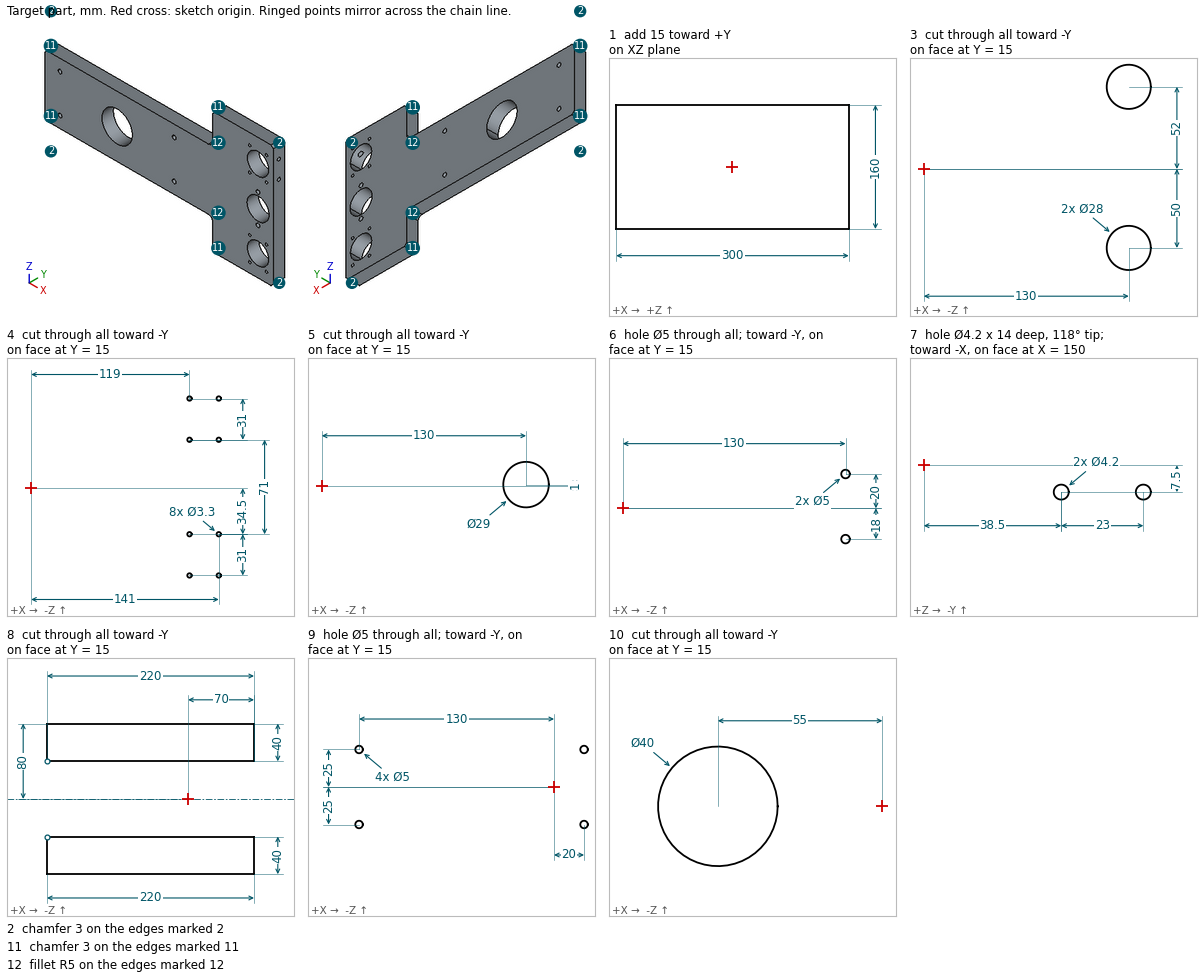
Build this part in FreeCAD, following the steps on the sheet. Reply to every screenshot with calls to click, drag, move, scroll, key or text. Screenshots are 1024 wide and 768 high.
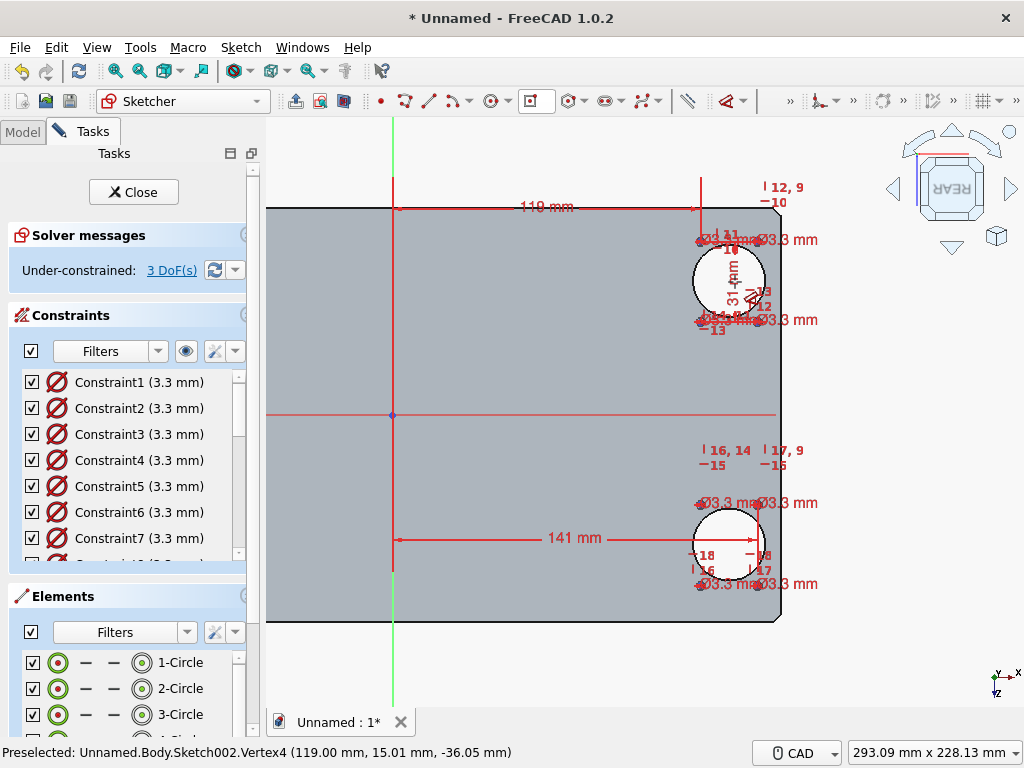
click(758, 505)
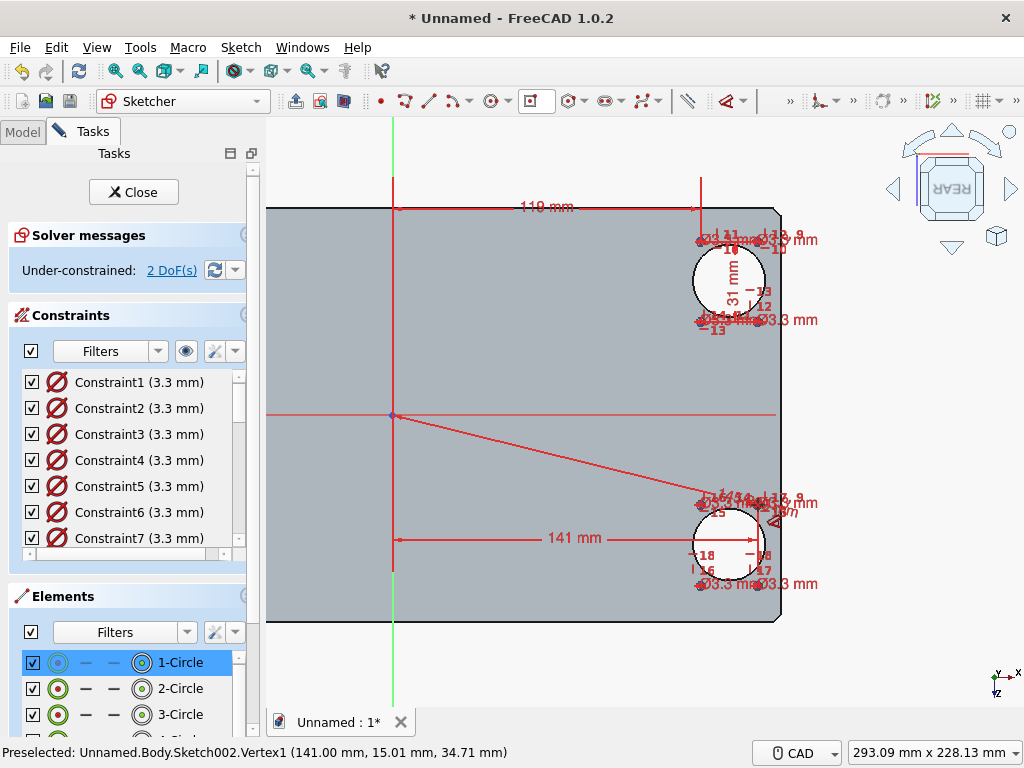
click(701, 322)
click(792, 371)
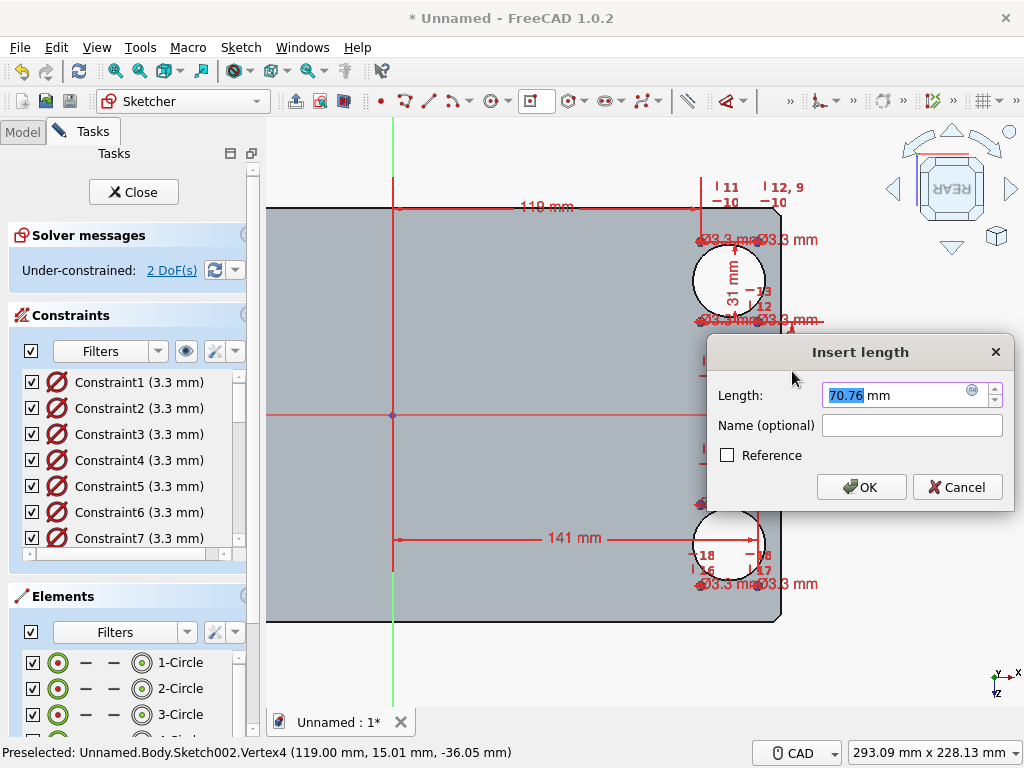
text(71)
key(Return)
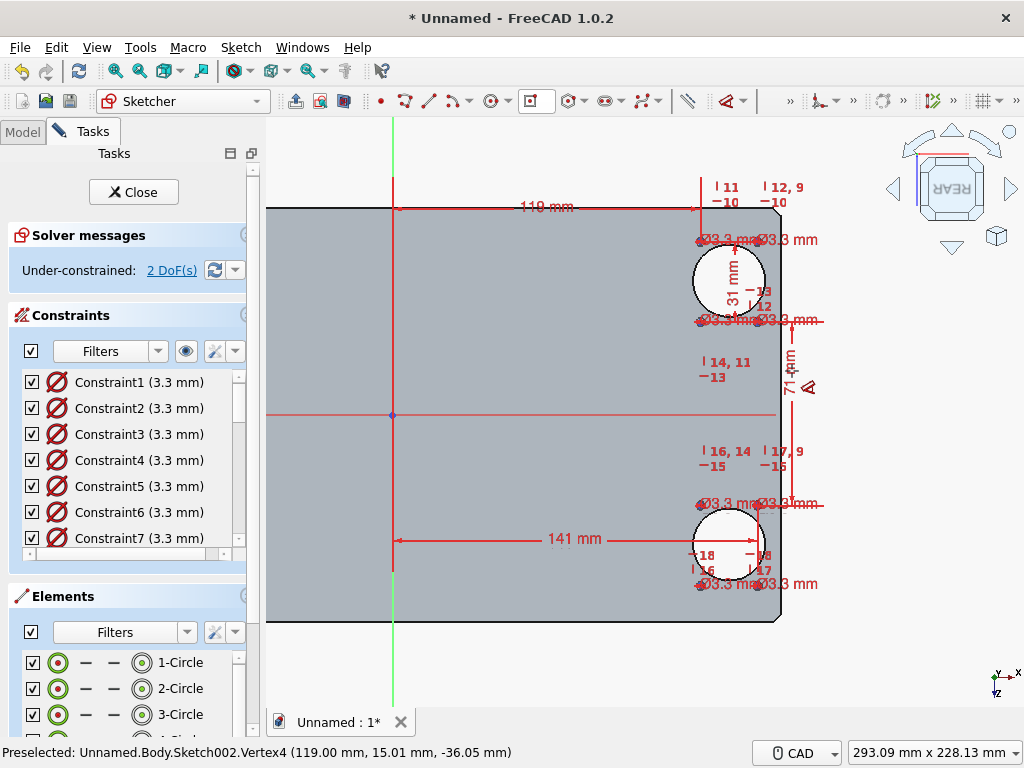
click(701, 506)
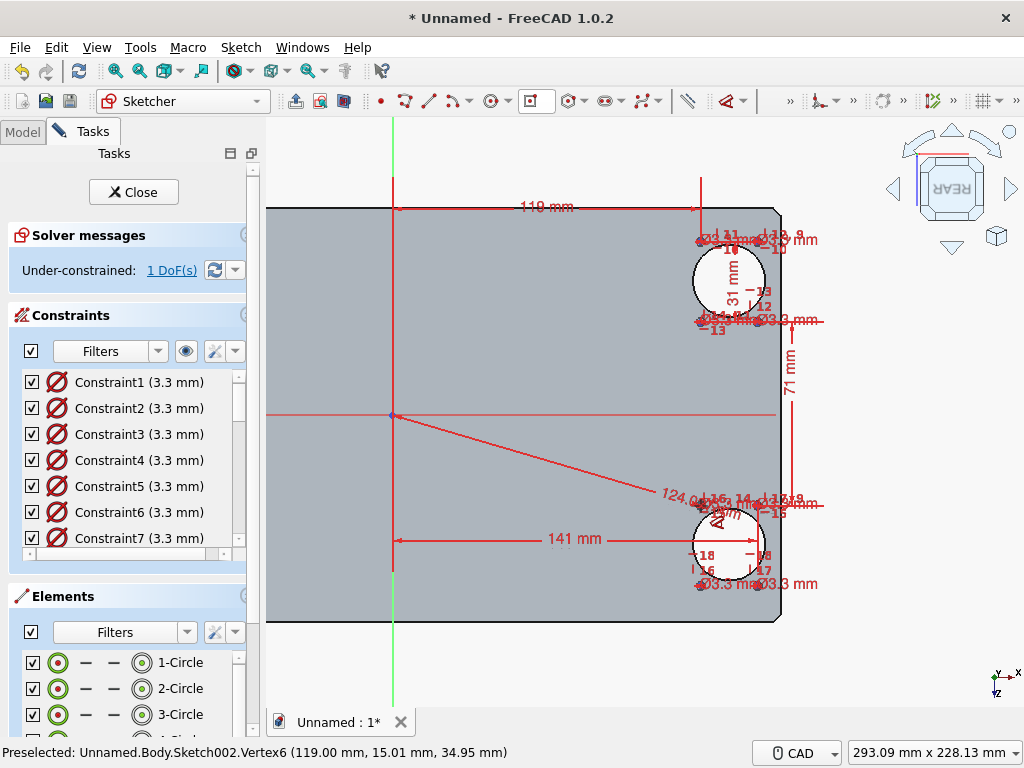
click(701, 586)
click(735, 546)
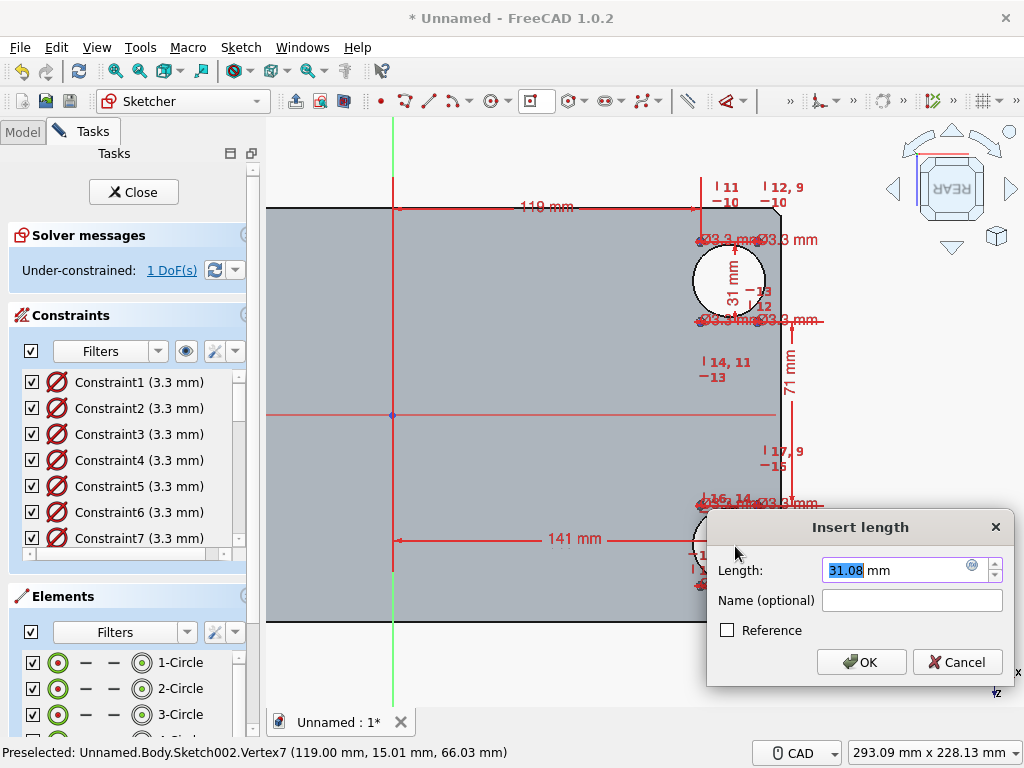
text(31)
key(Return)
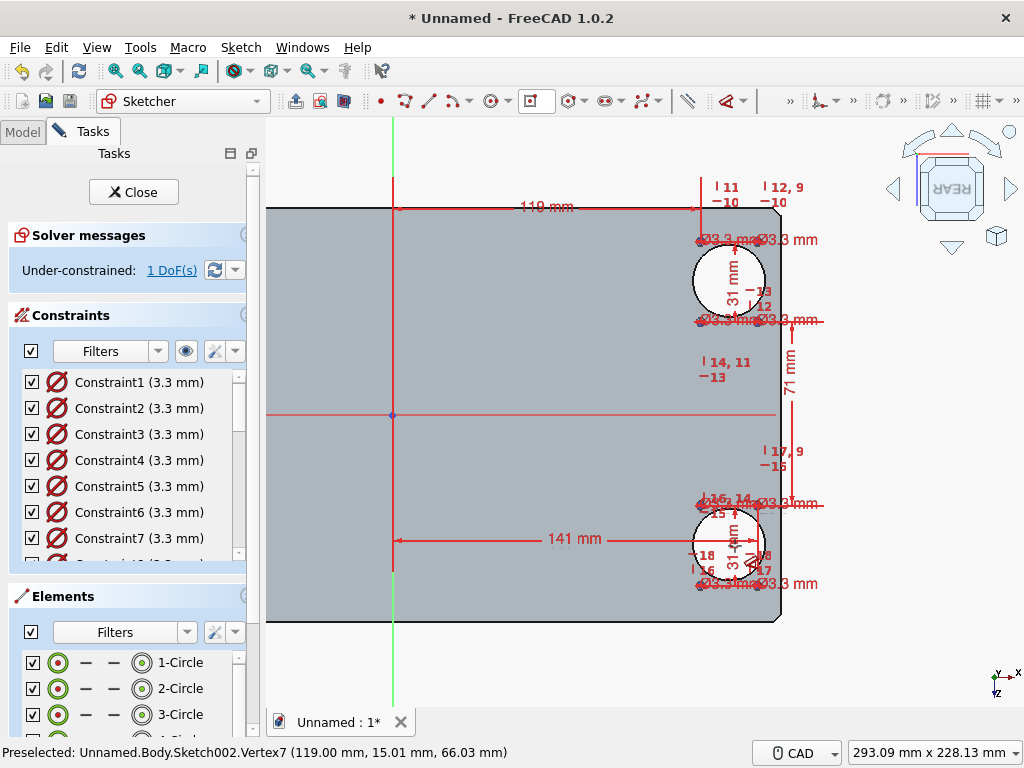
click(758, 506)
click(359, 460)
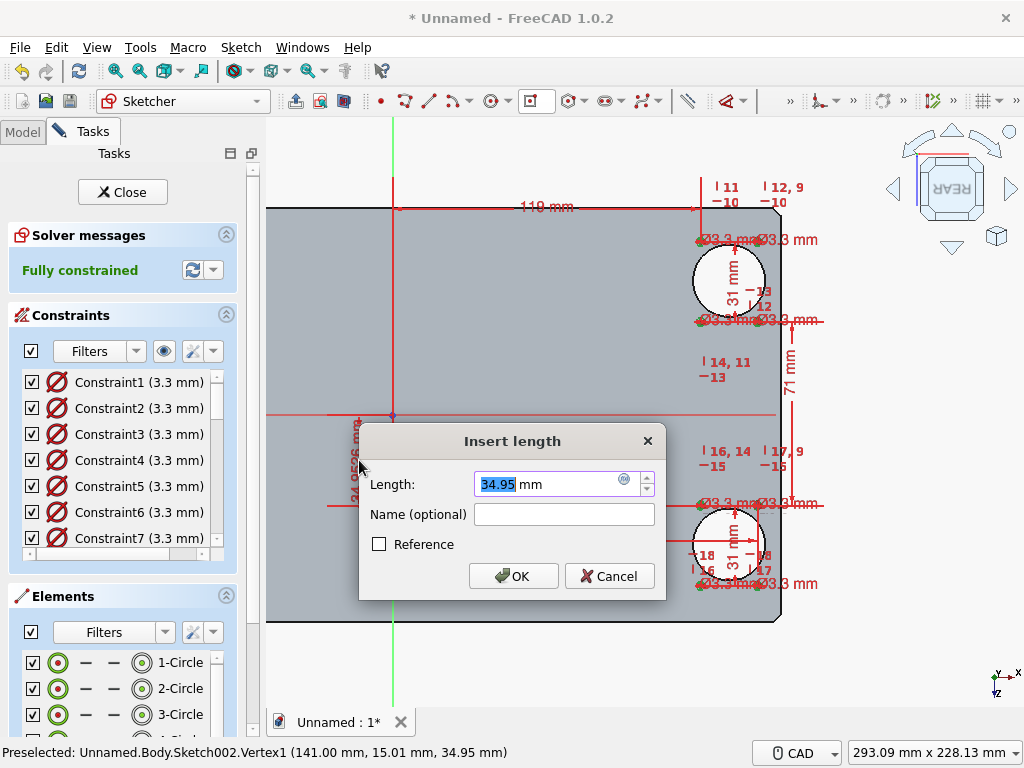
text(34.5)
key(Return)
key(Escape)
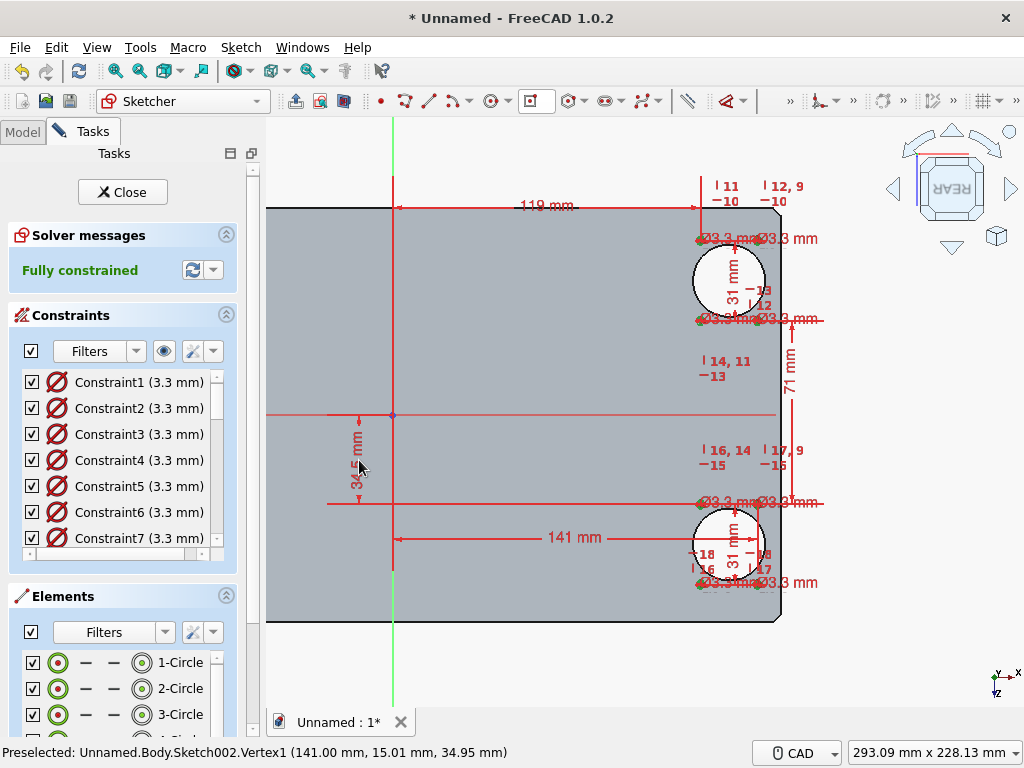
click(123, 192)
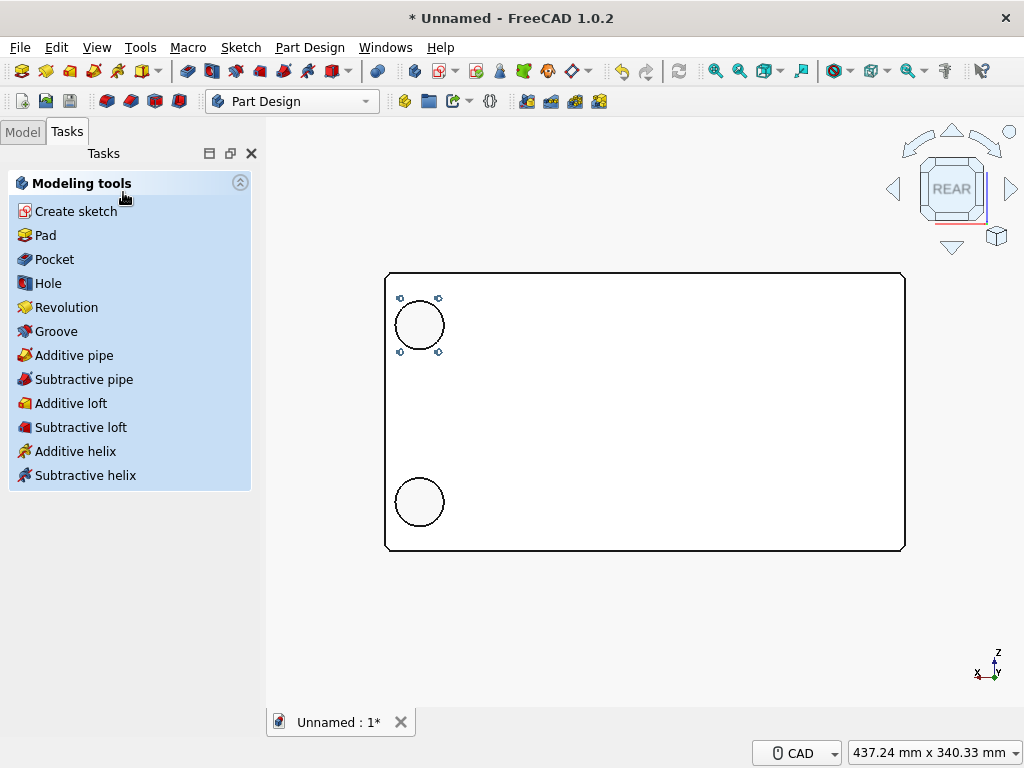
click(188, 72)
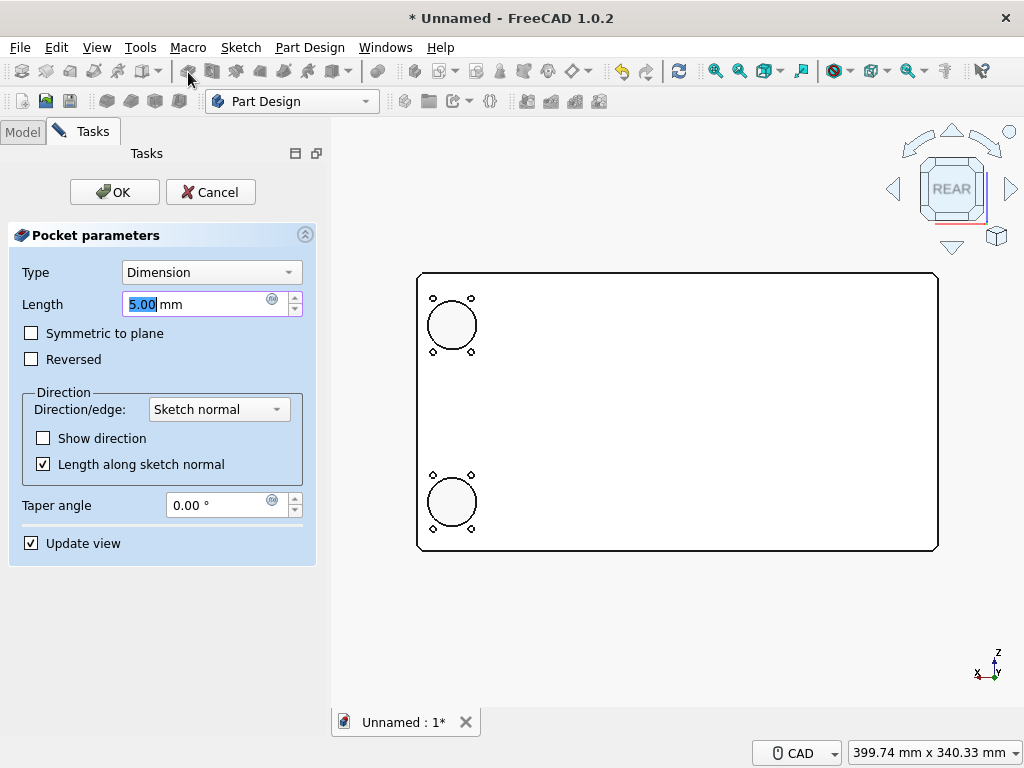
click(212, 272)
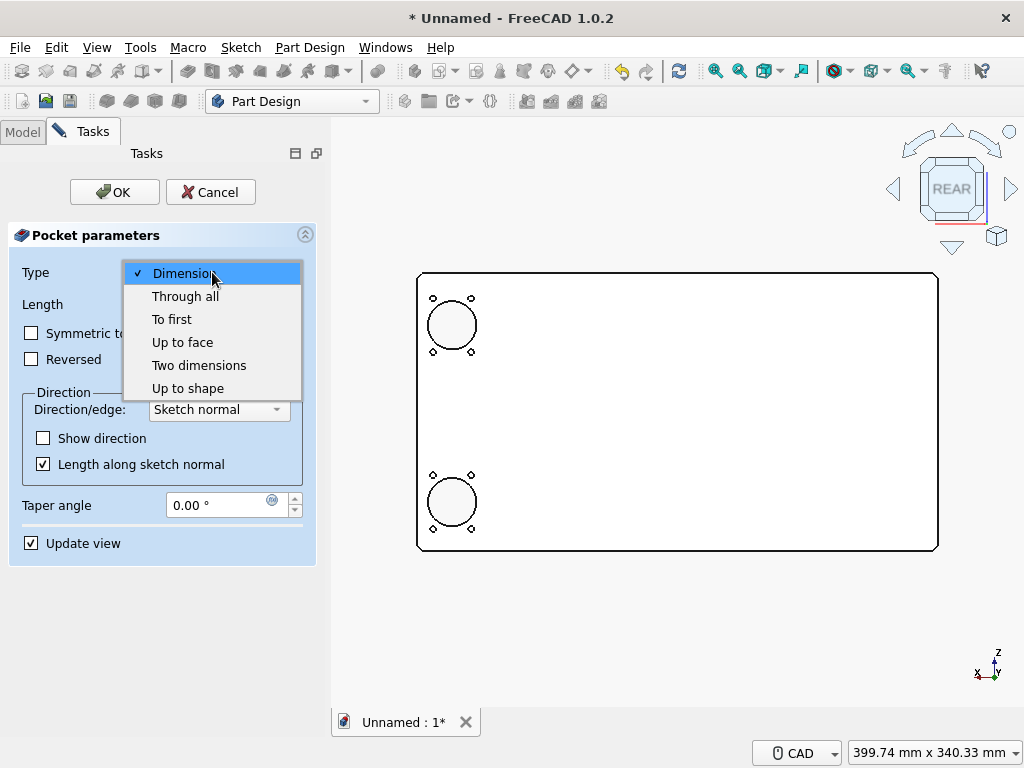
click(212, 296)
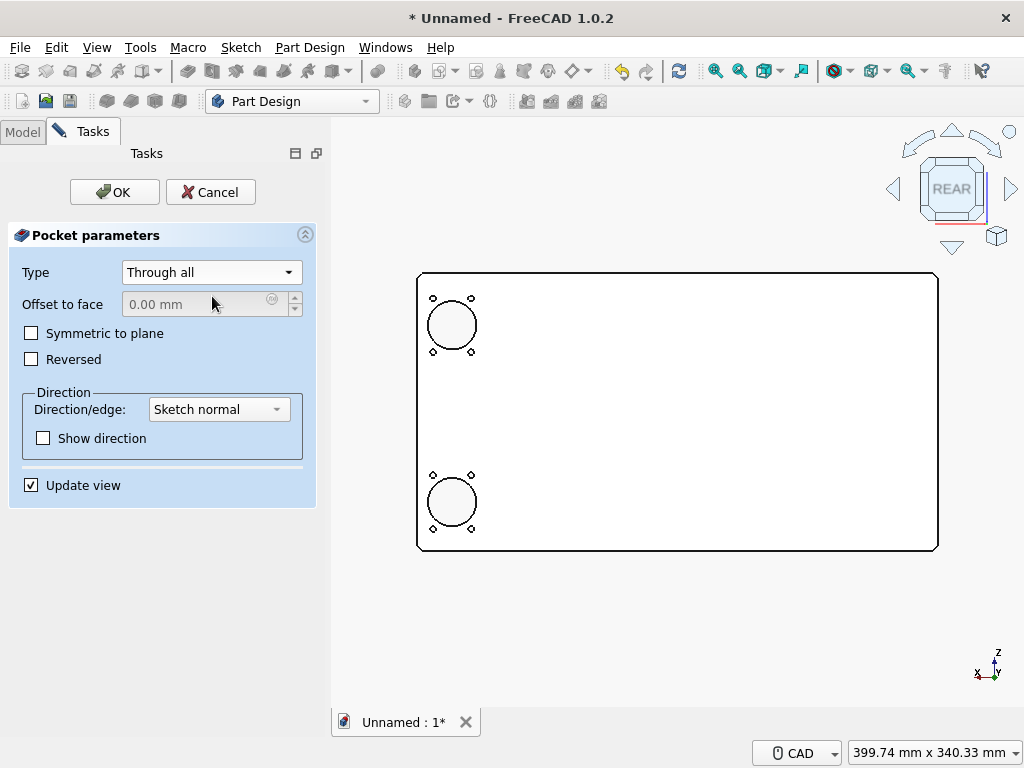
click(115, 192)